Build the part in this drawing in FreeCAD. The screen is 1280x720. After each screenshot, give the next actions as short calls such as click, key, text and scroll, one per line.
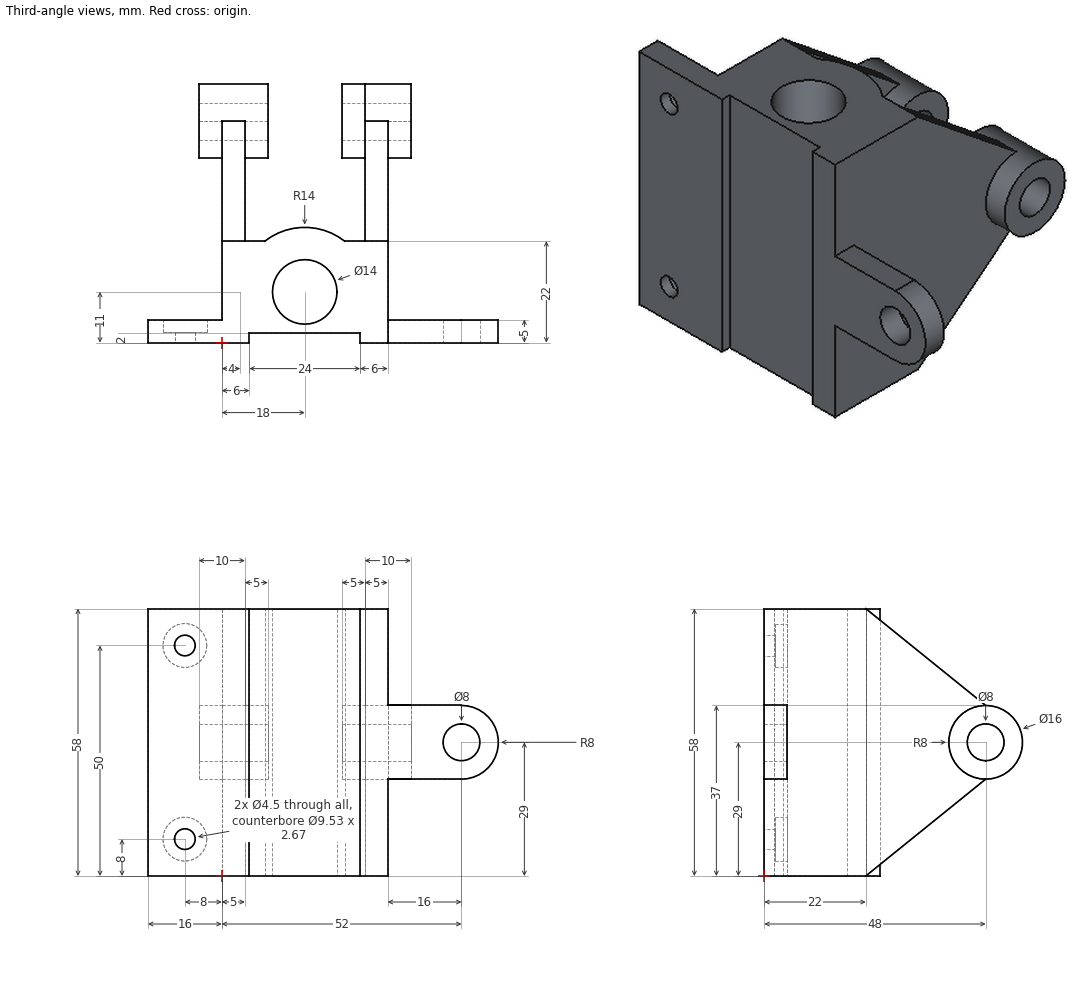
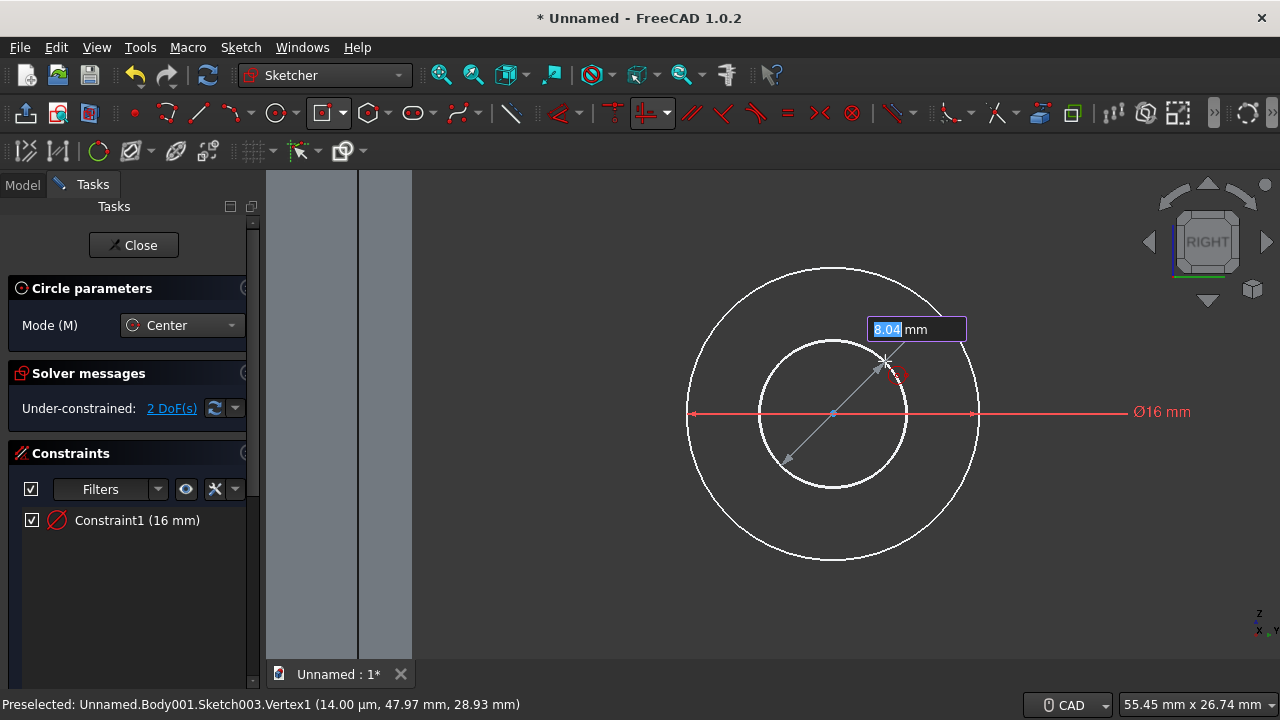
text(8)
key(Return)
key(Escape)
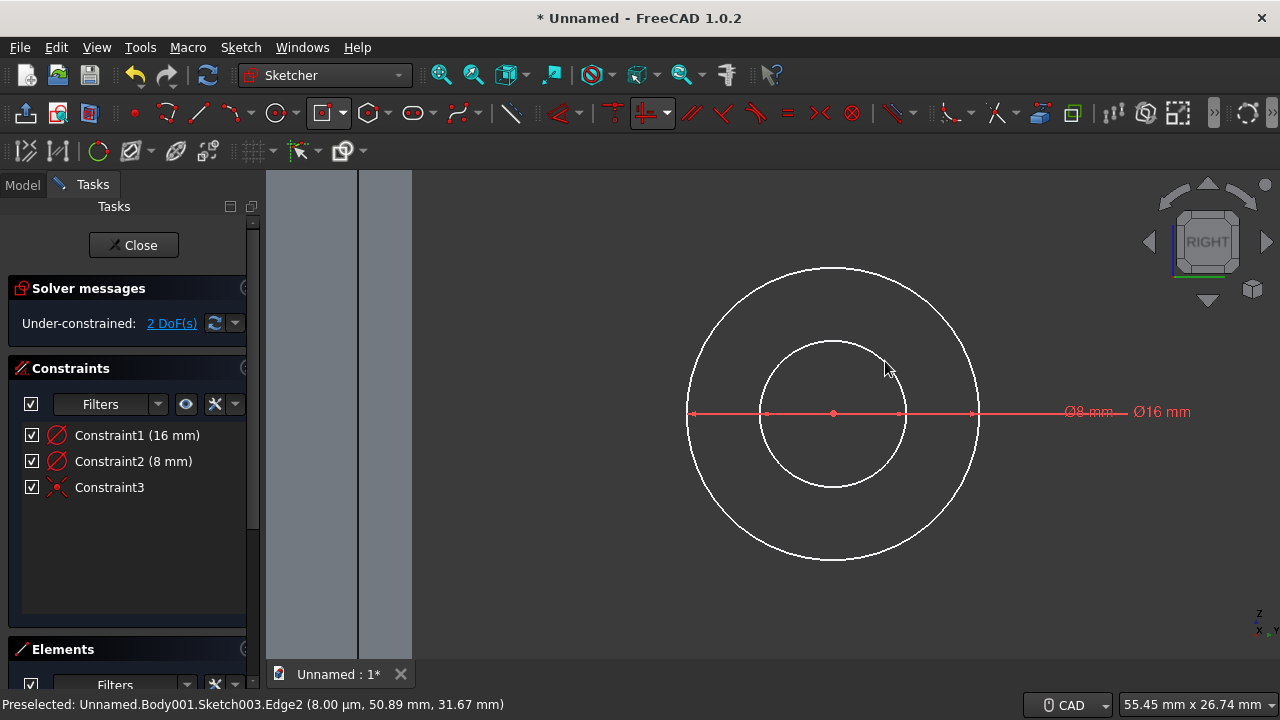
key(d)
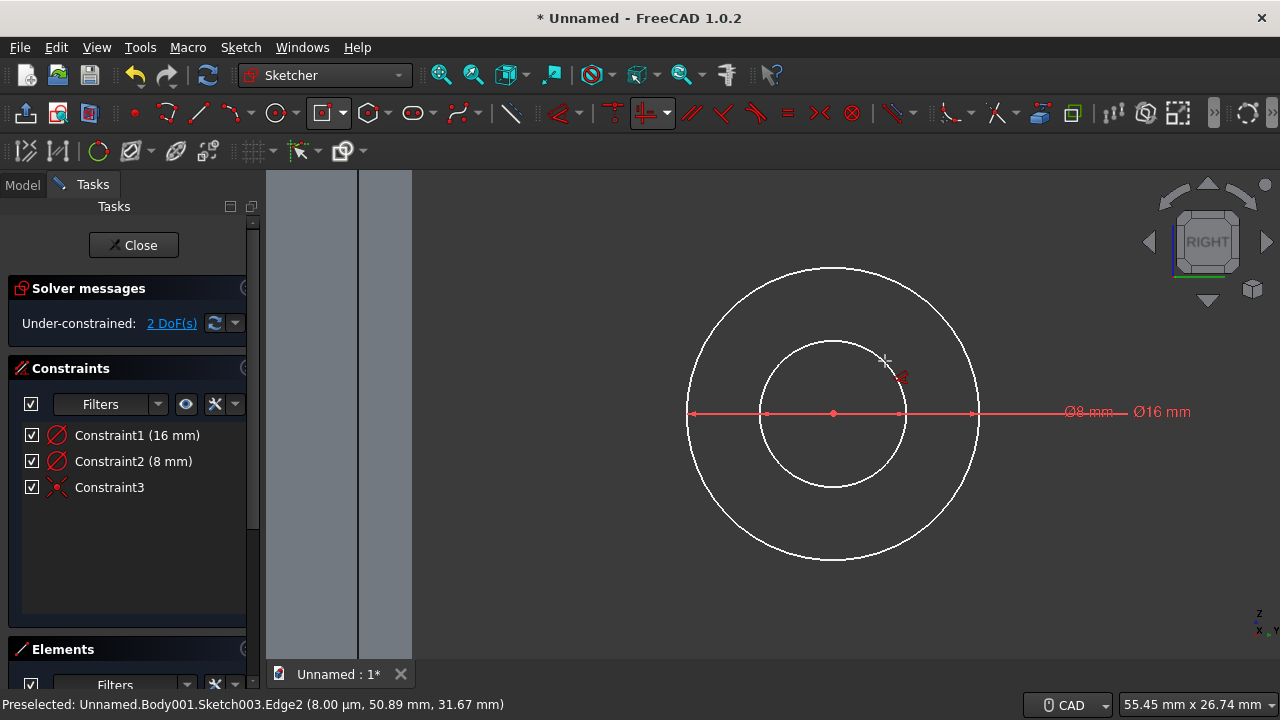
click(833, 414)
click(564, 380)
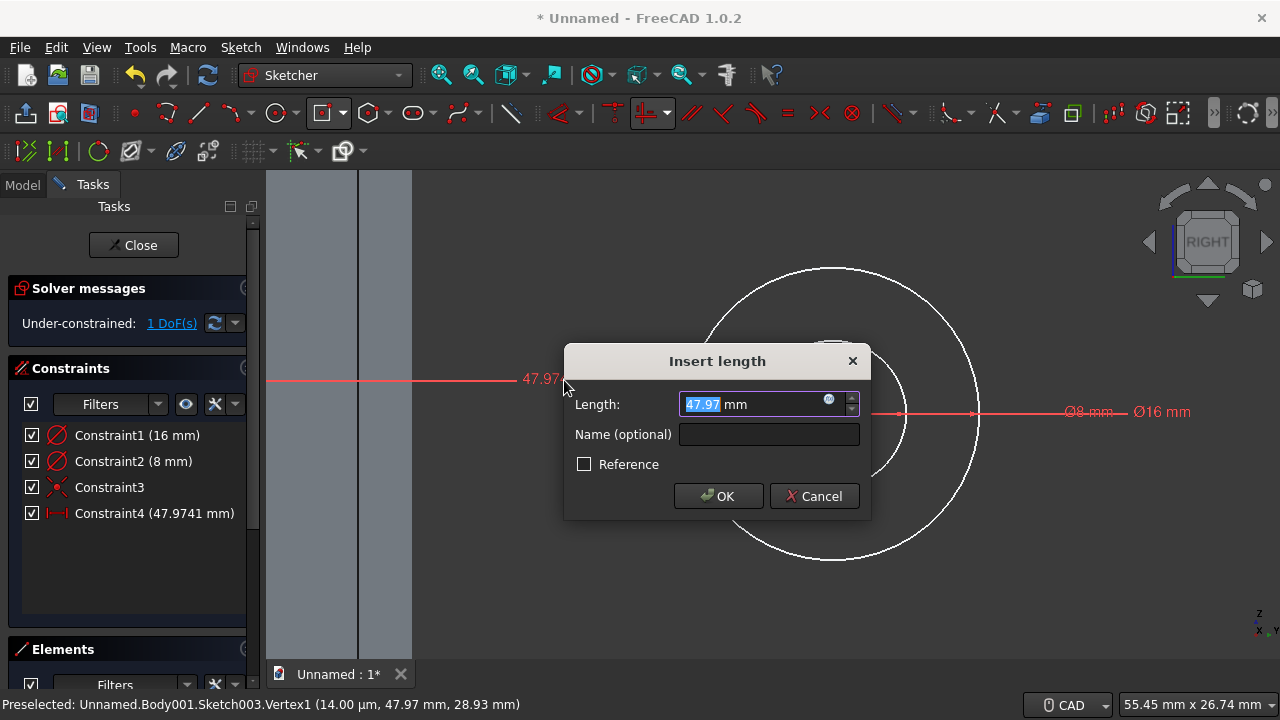
text(48)
key(Return)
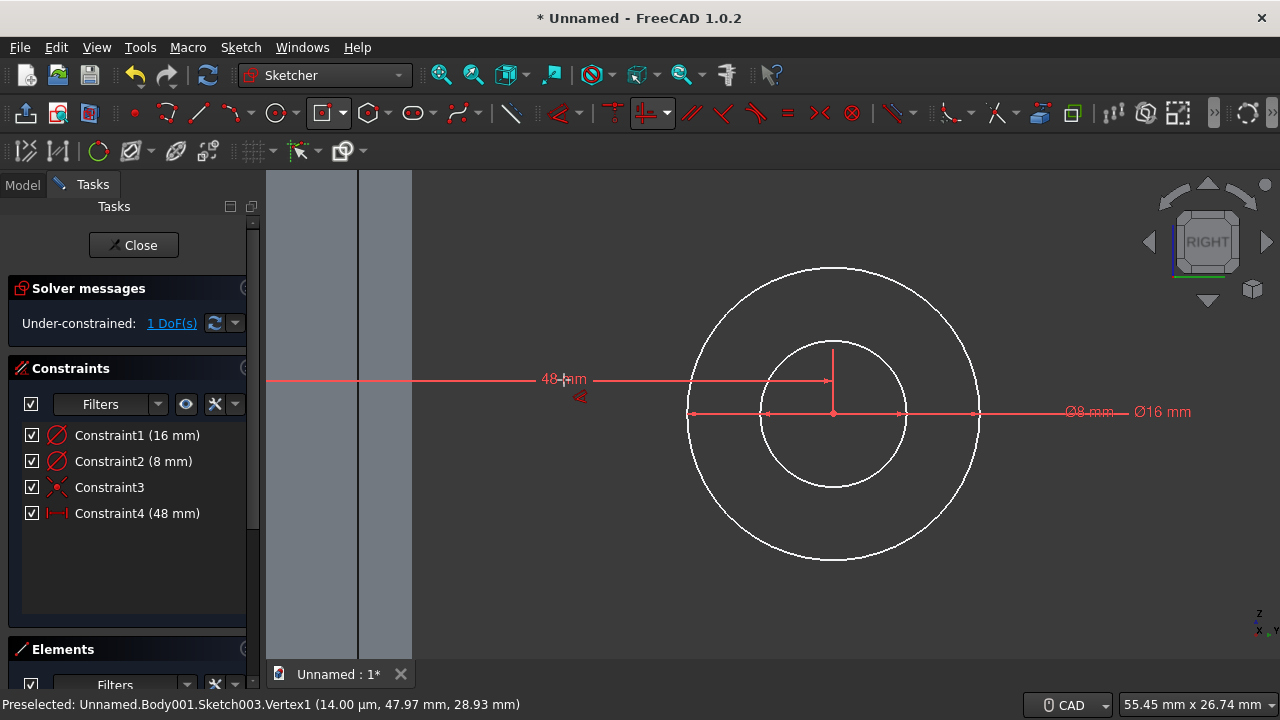
click(833, 414)
click(867, 522)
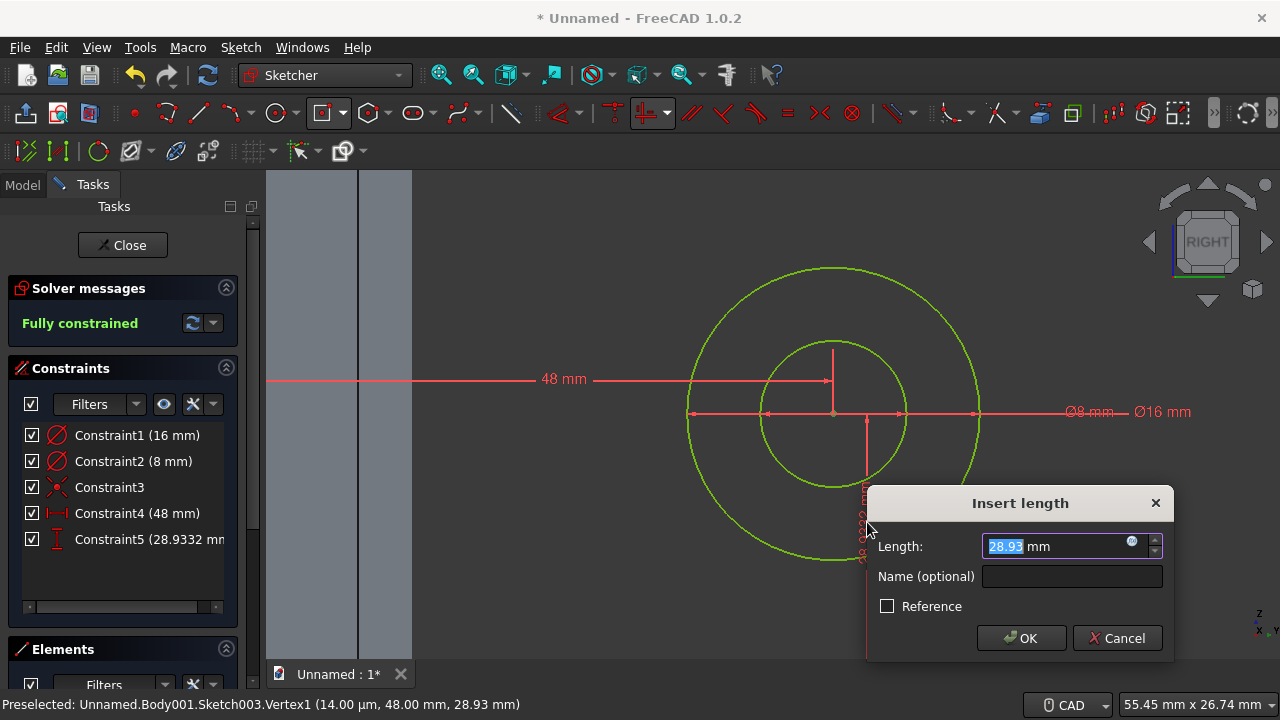
text(29)
key(Return)
key(Escape)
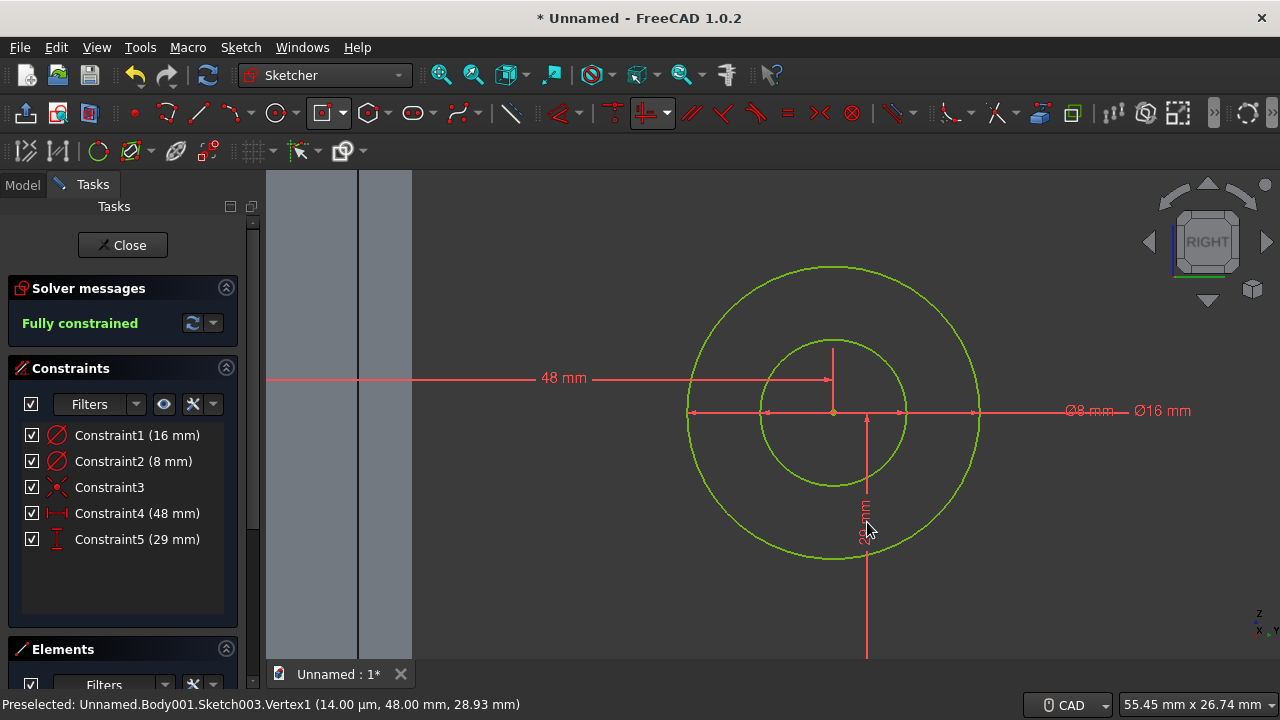
click(123, 245)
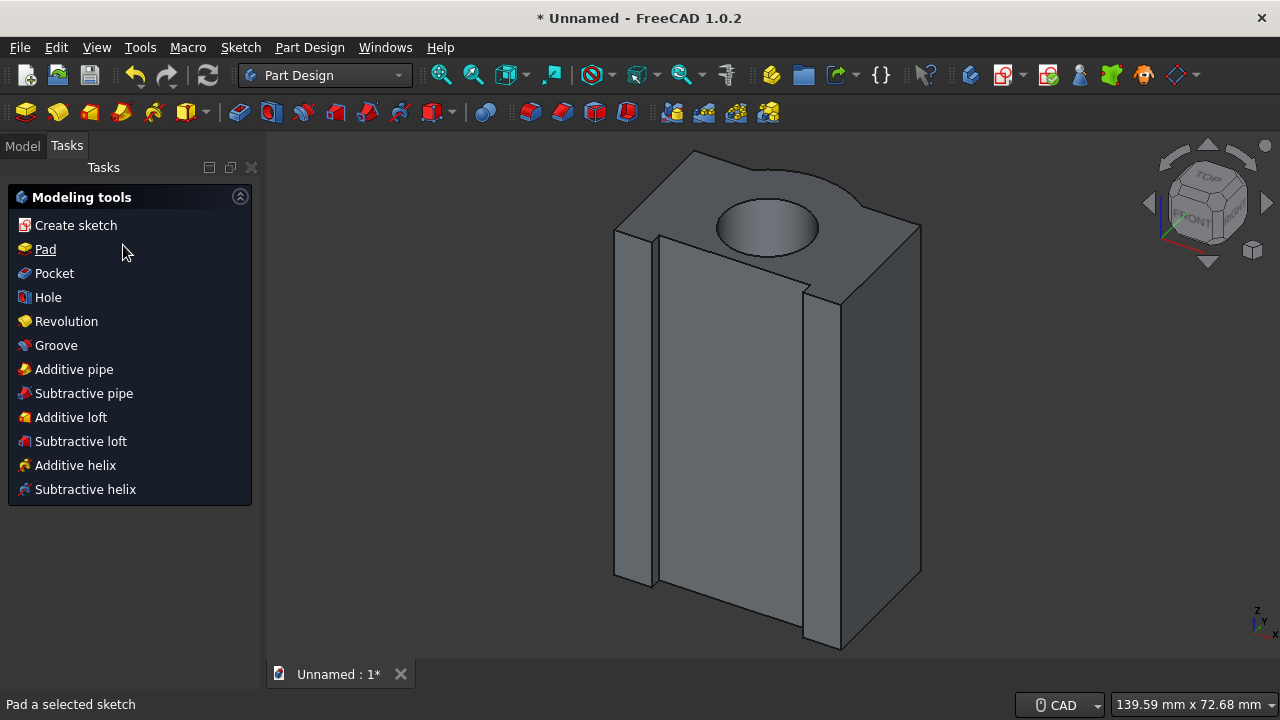
click(26, 112)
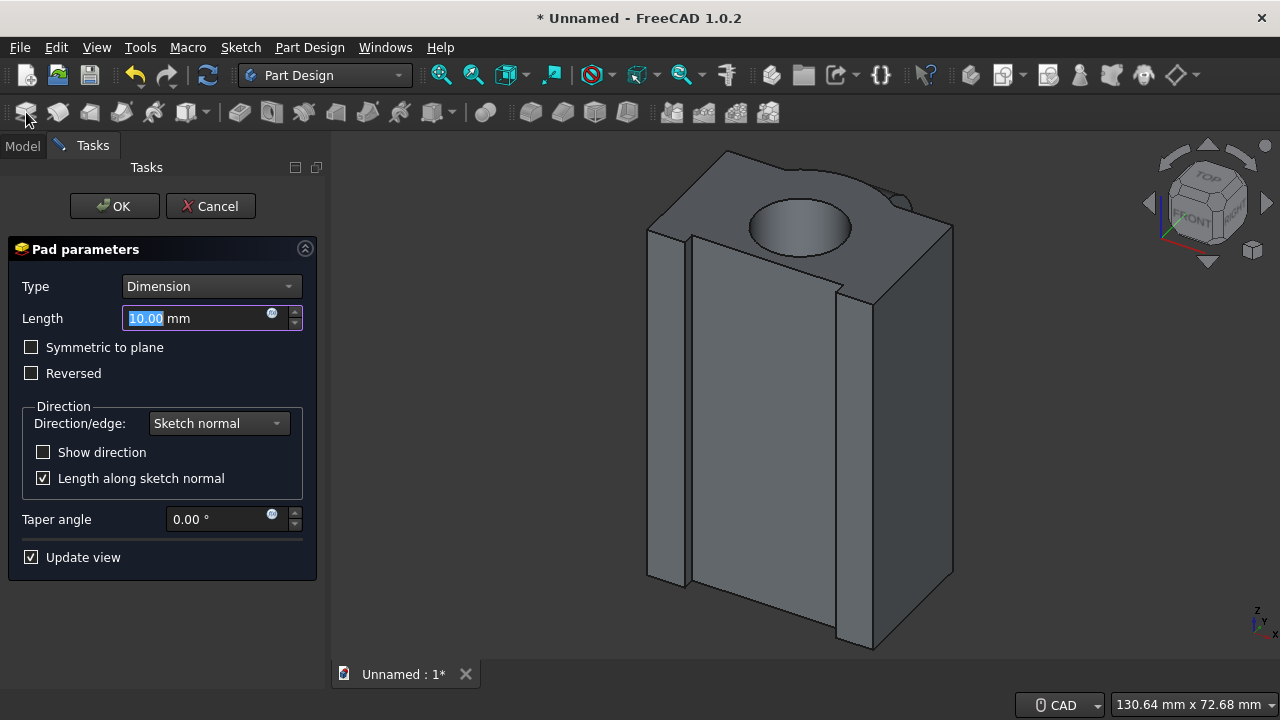
text(10)
key(Tab)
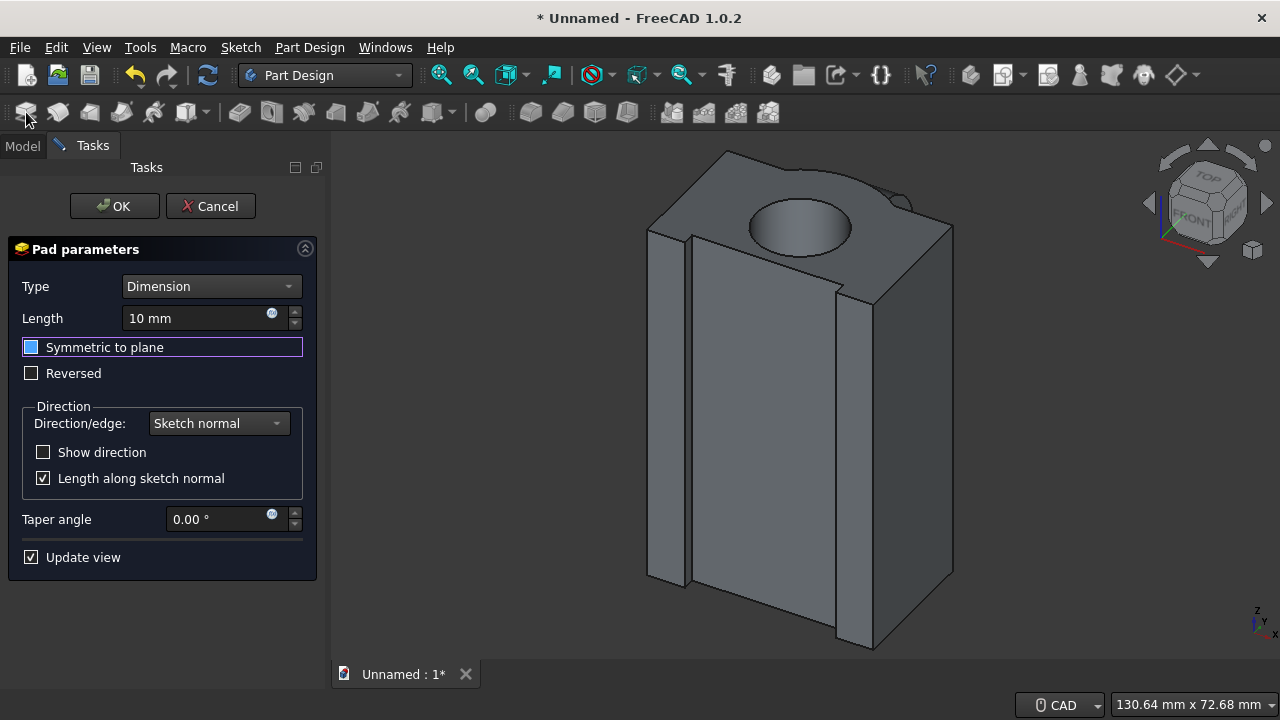
click(30, 347)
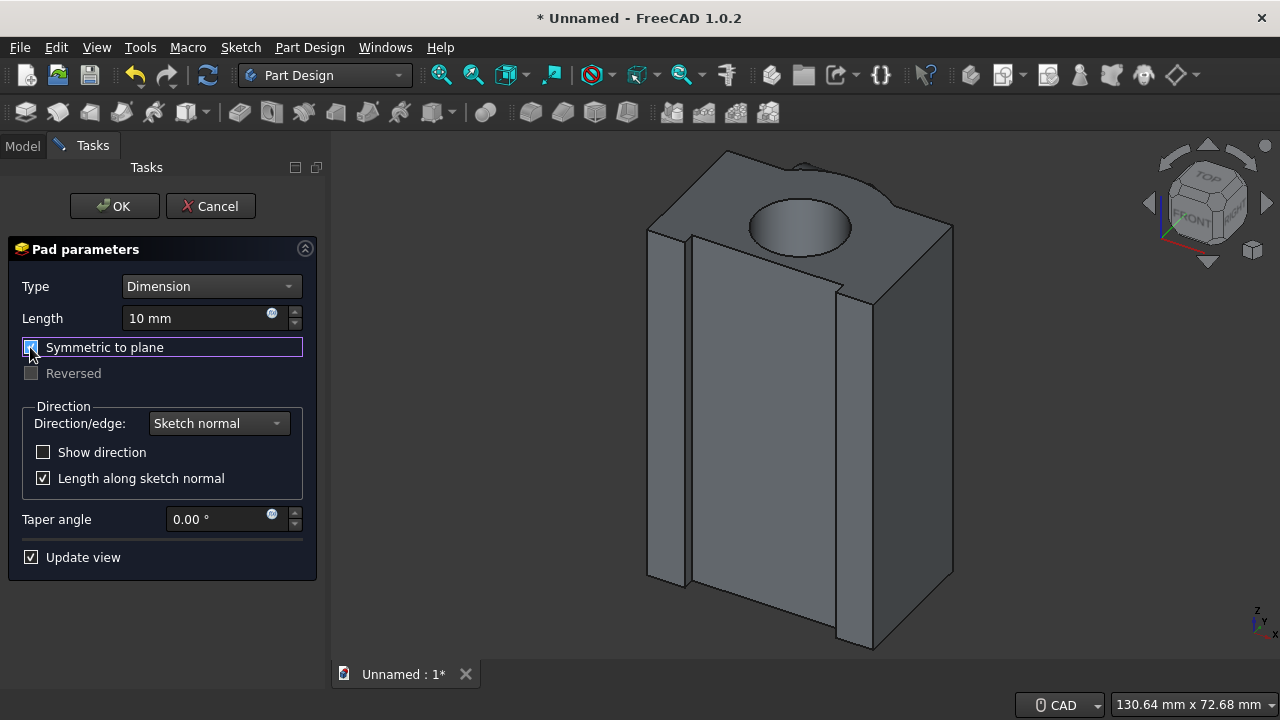
click(115, 206)